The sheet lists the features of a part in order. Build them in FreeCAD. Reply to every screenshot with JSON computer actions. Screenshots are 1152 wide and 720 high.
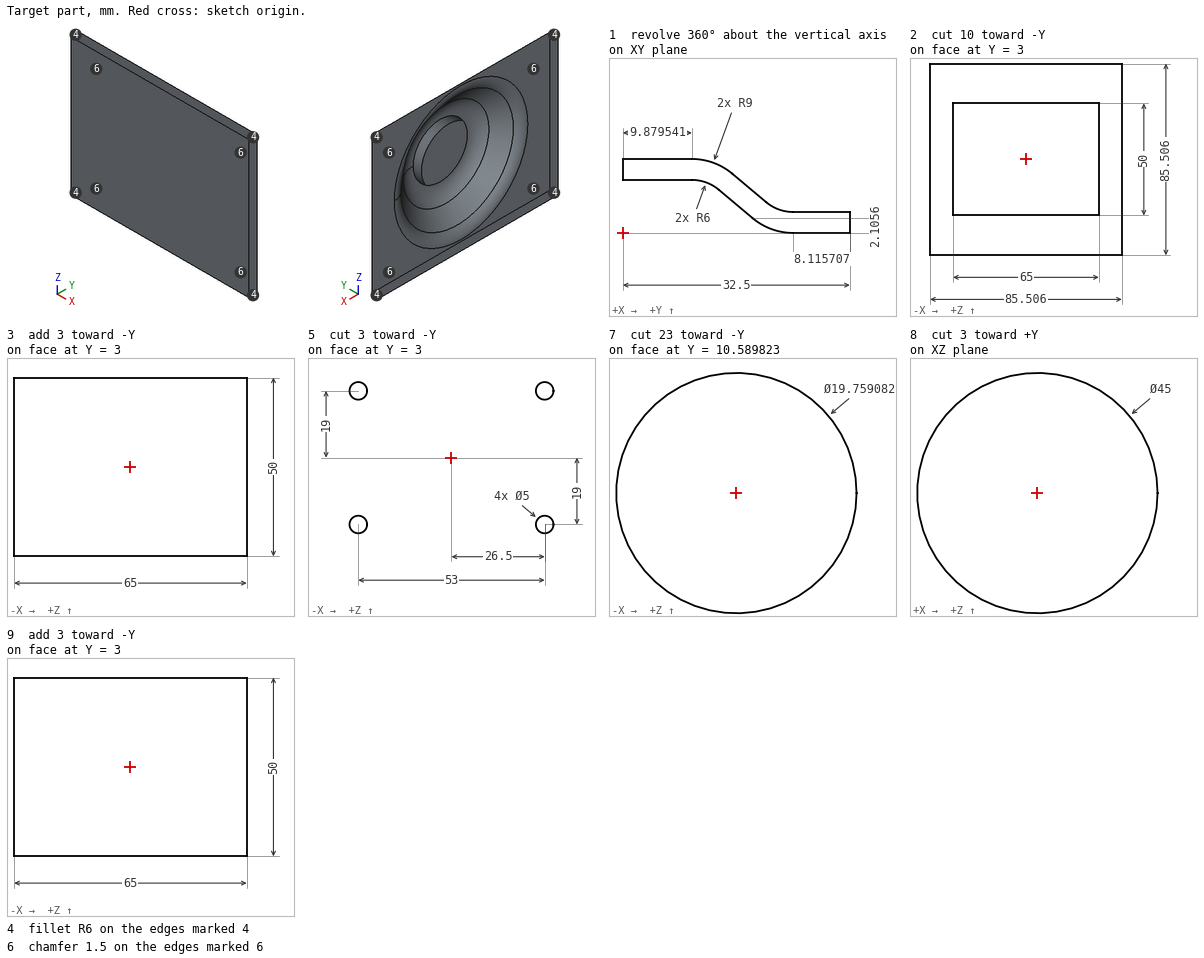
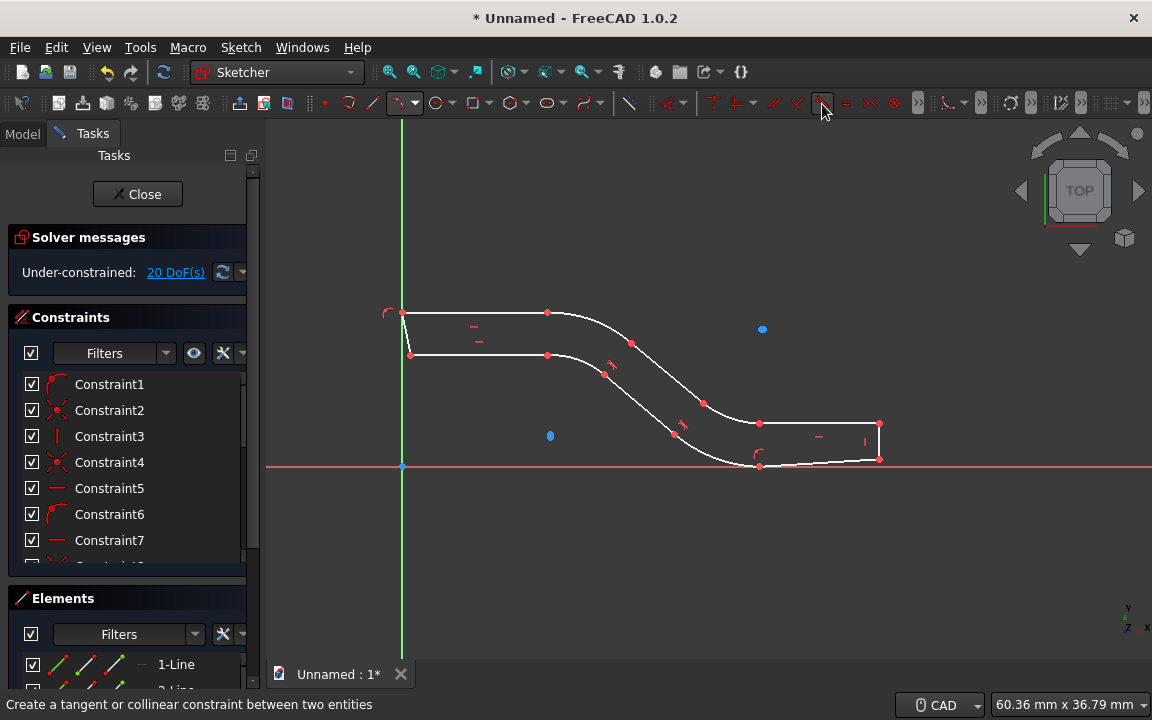
{"action": "left_click", "coordinate": [795, 465]}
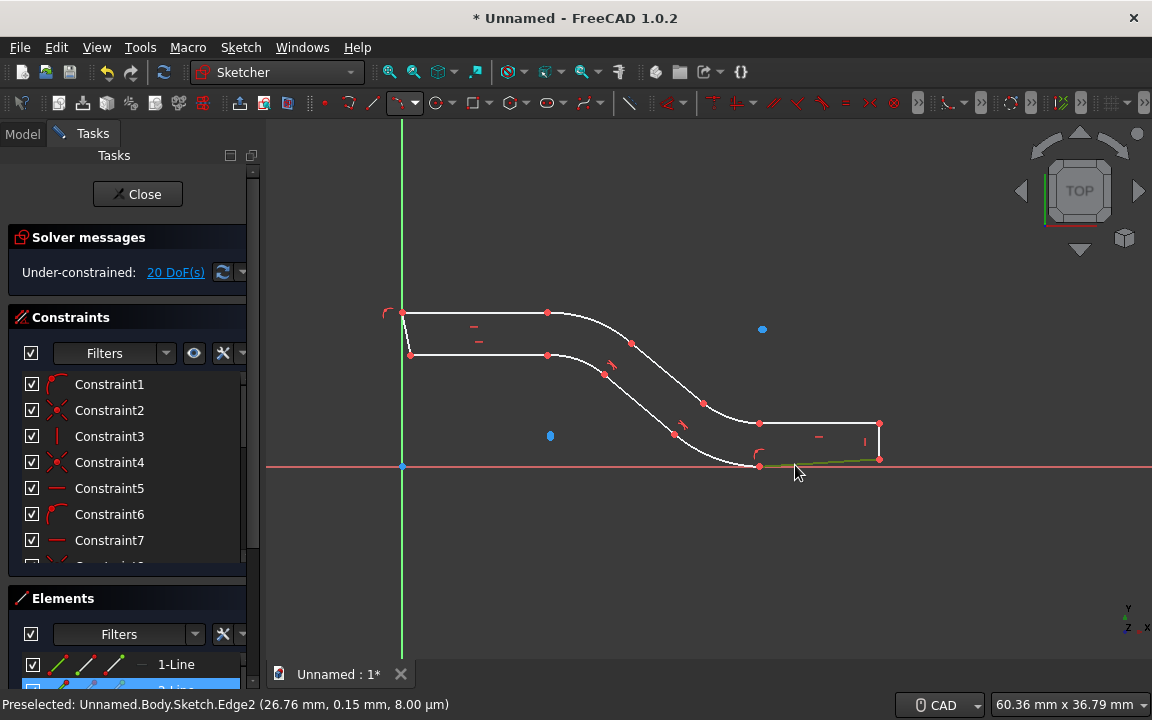
{"action": "left_click", "coordinate": [698, 450]}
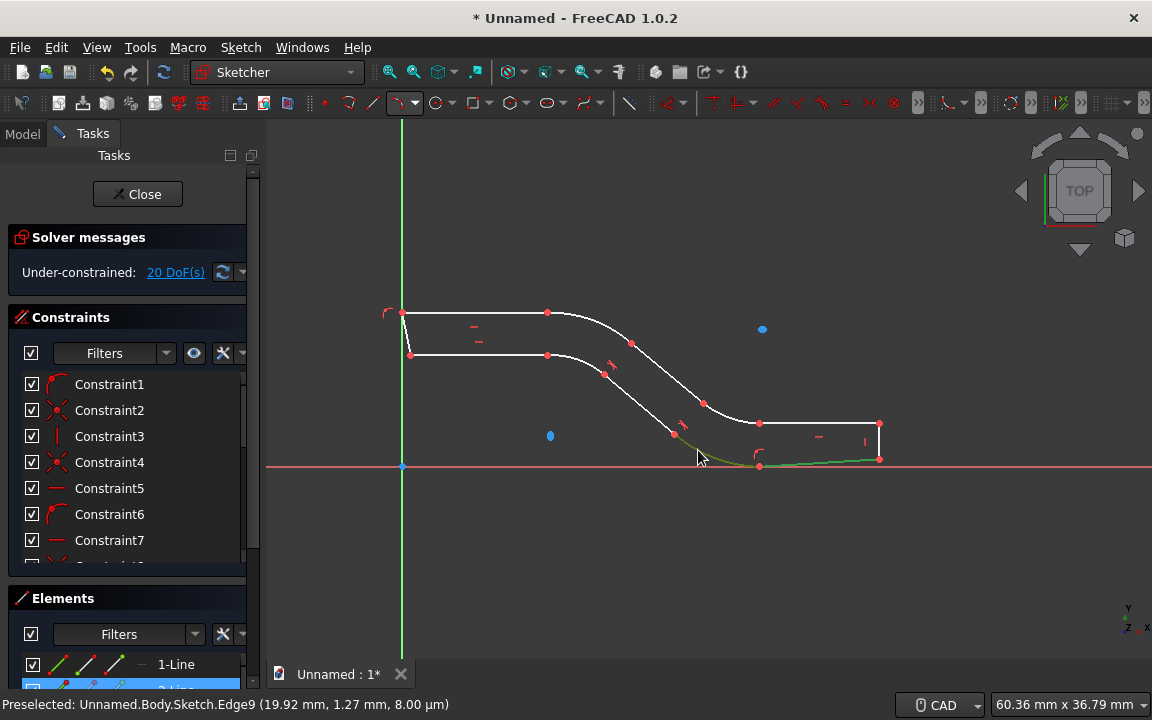
{"action": "left_click", "coordinate": [822, 104]}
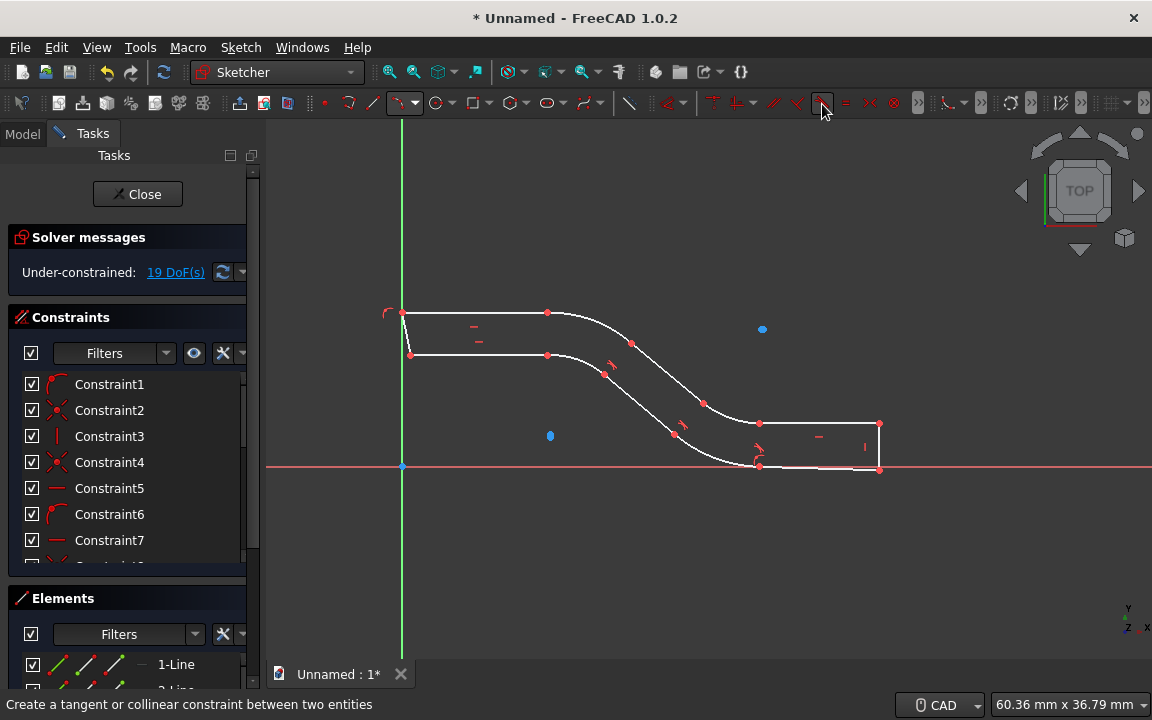
{"action": "left_click", "coordinate": [843, 423]}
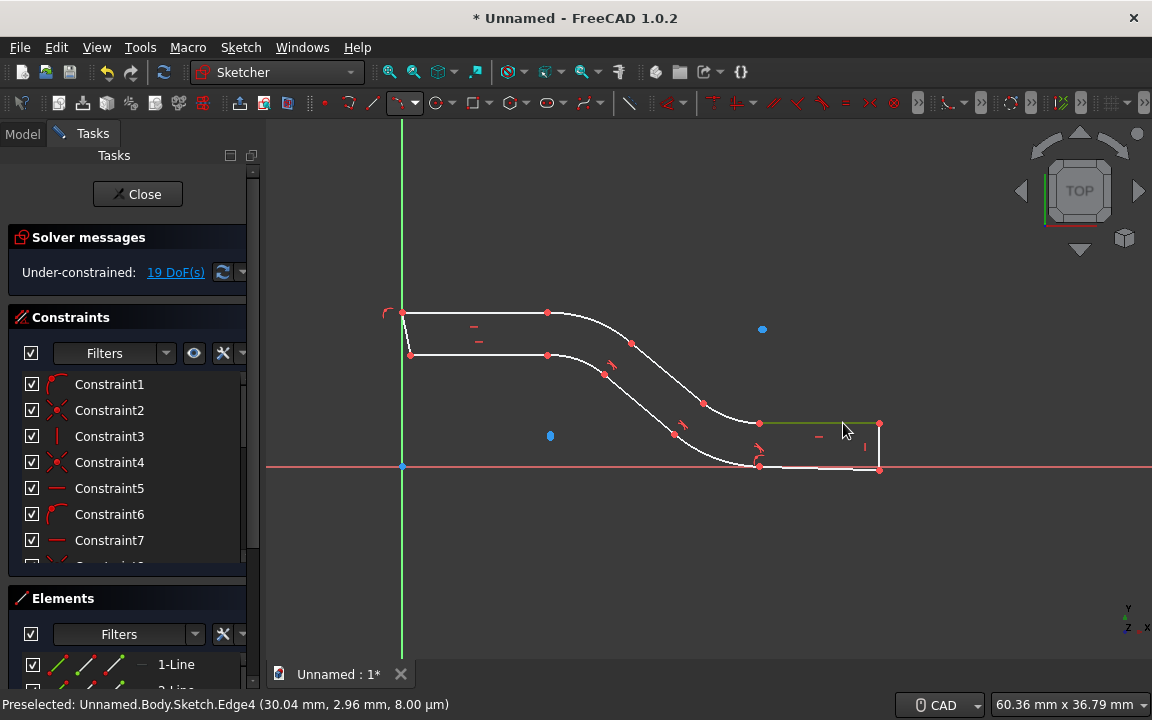
{"action": "left_click", "coordinate": [719, 413]}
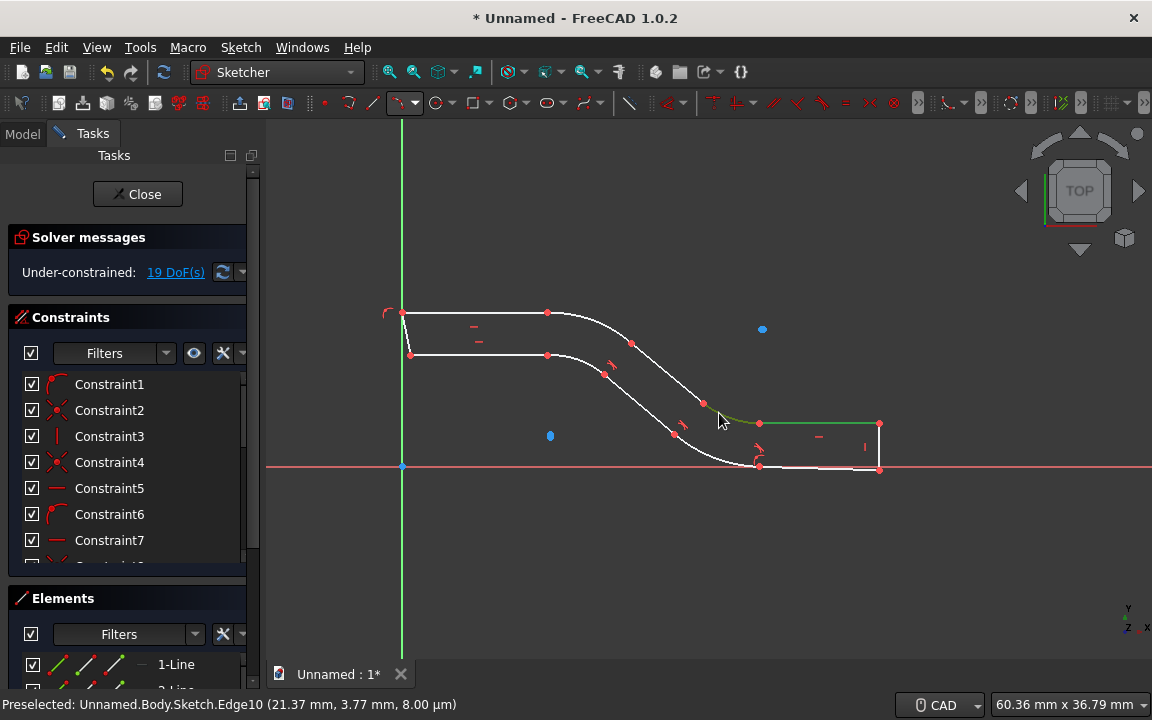
{"action": "left_click", "coordinate": [822, 104]}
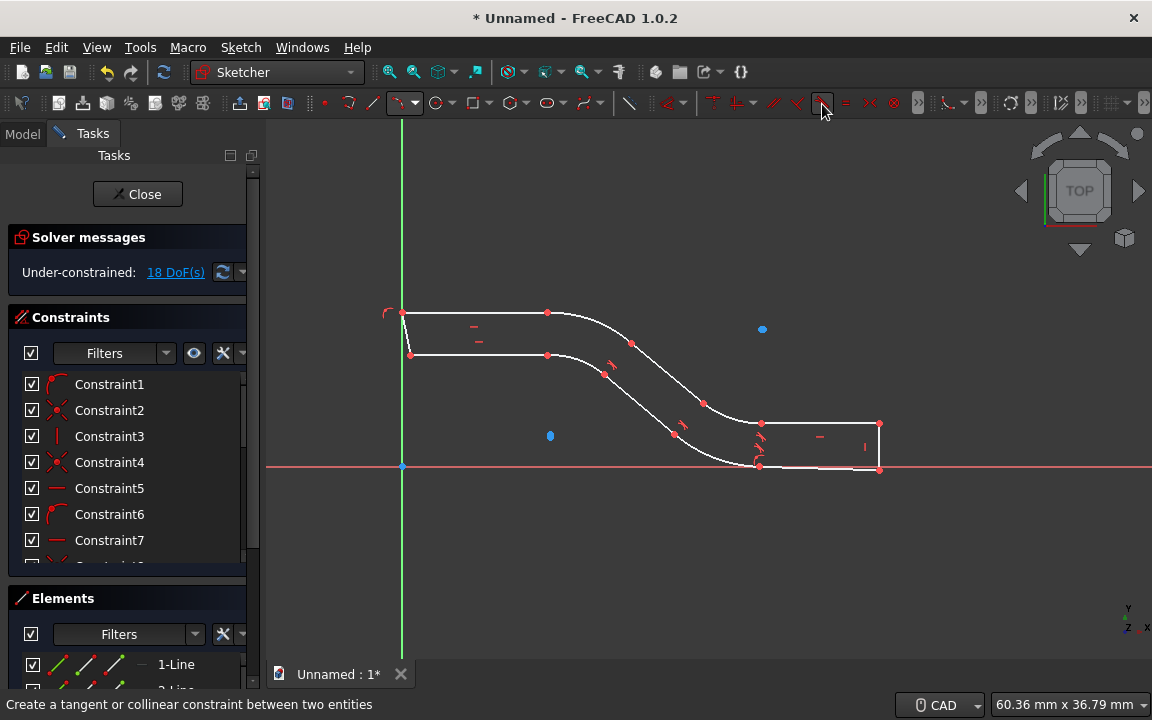
{"action": "left_click", "coordinate": [682, 386]}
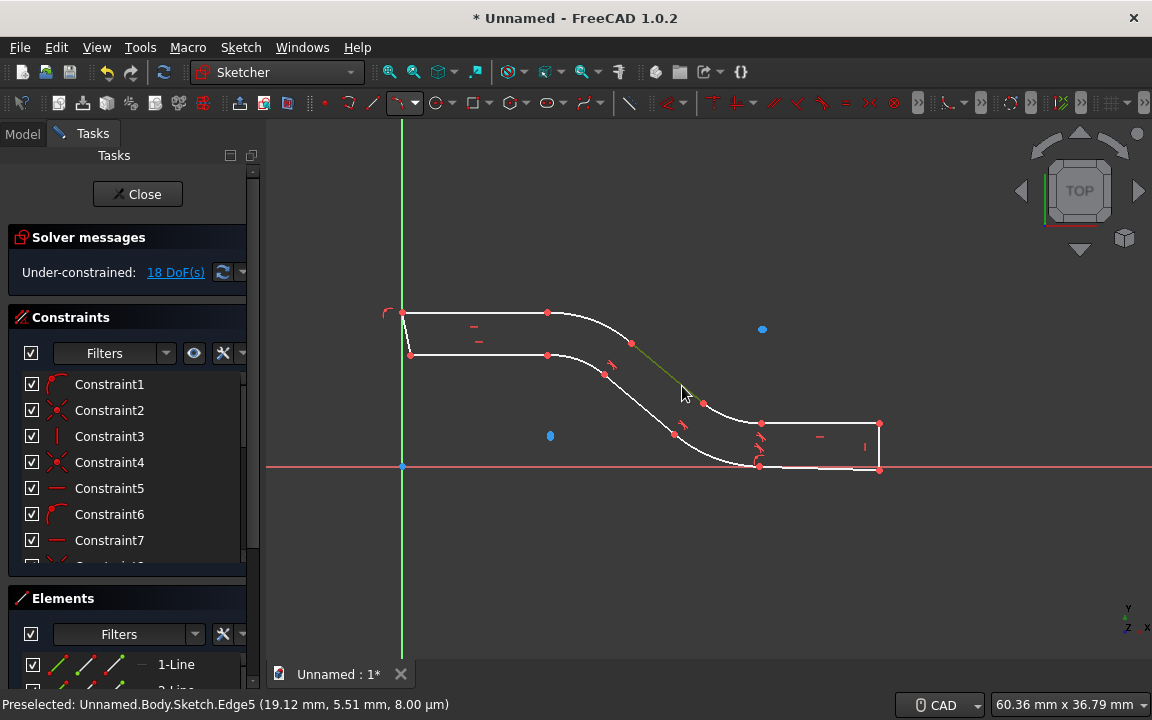
{"action": "left_click", "coordinate": [720, 413]}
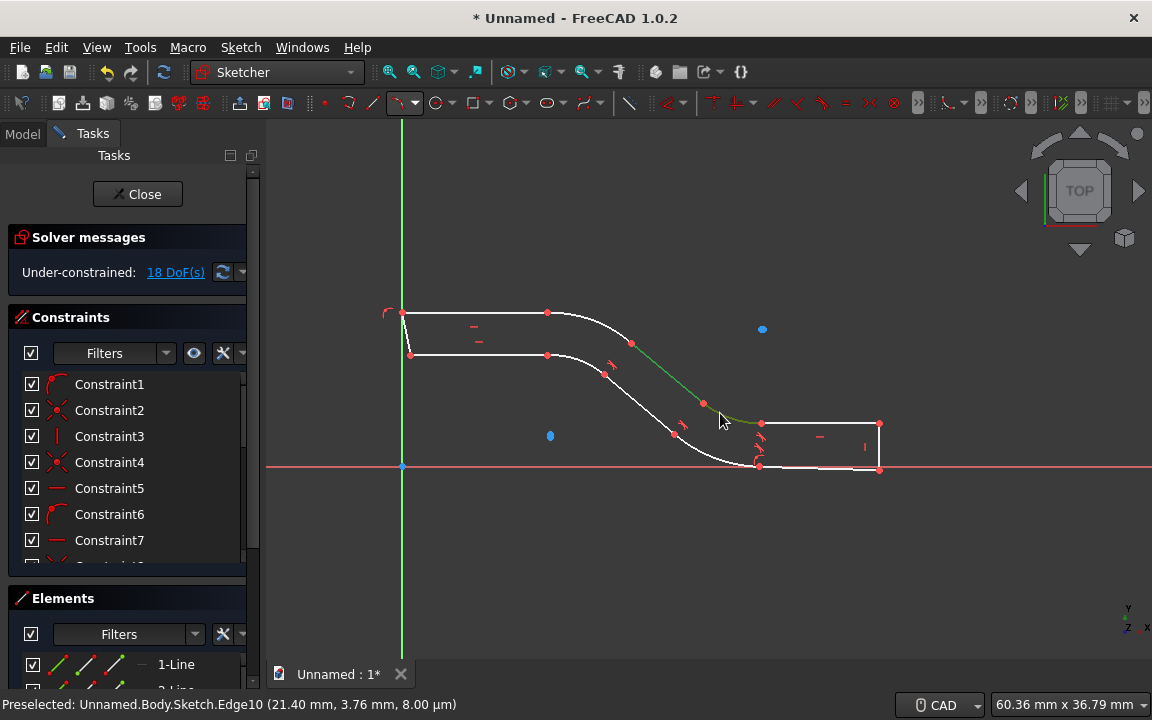
{"action": "left_click", "coordinate": [822, 104]}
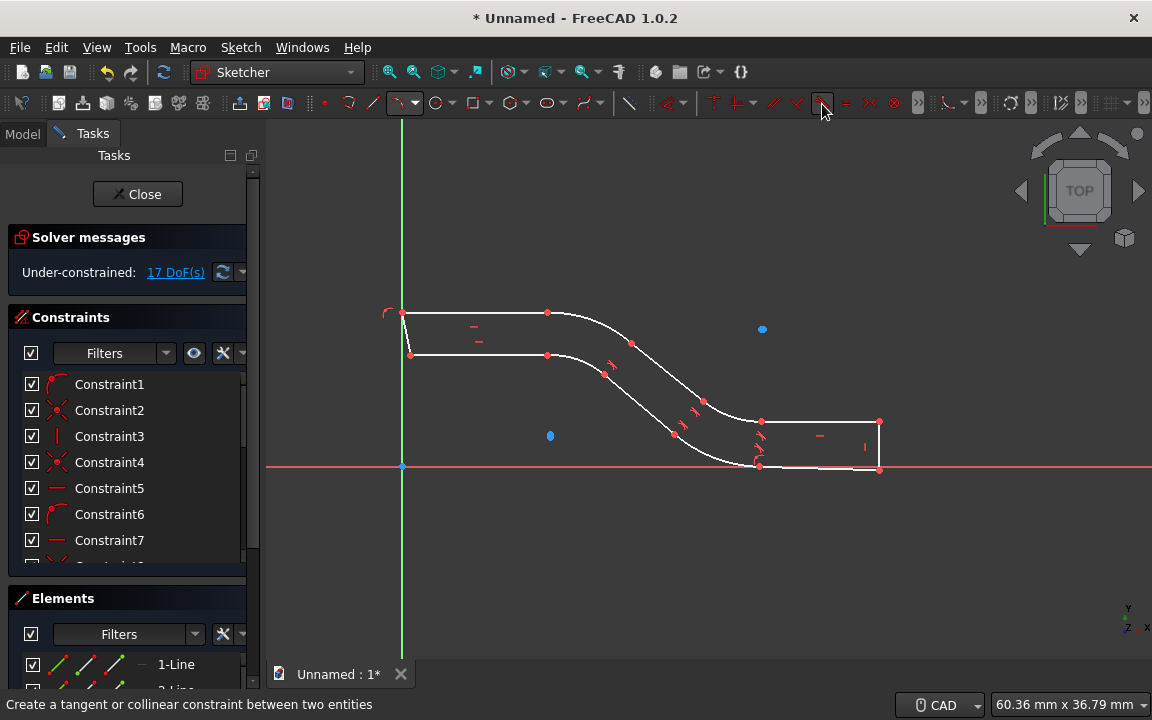
{"action": "left_click", "coordinate": [682, 384]}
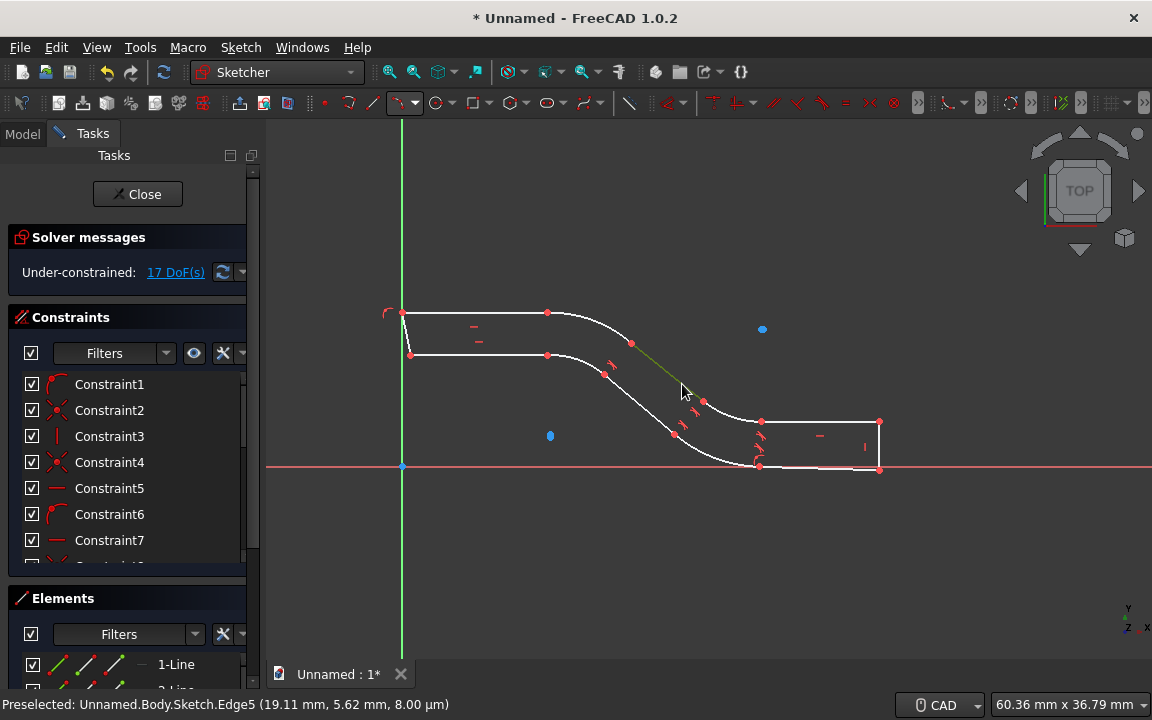
{"action": "left_click", "coordinate": [609, 328]}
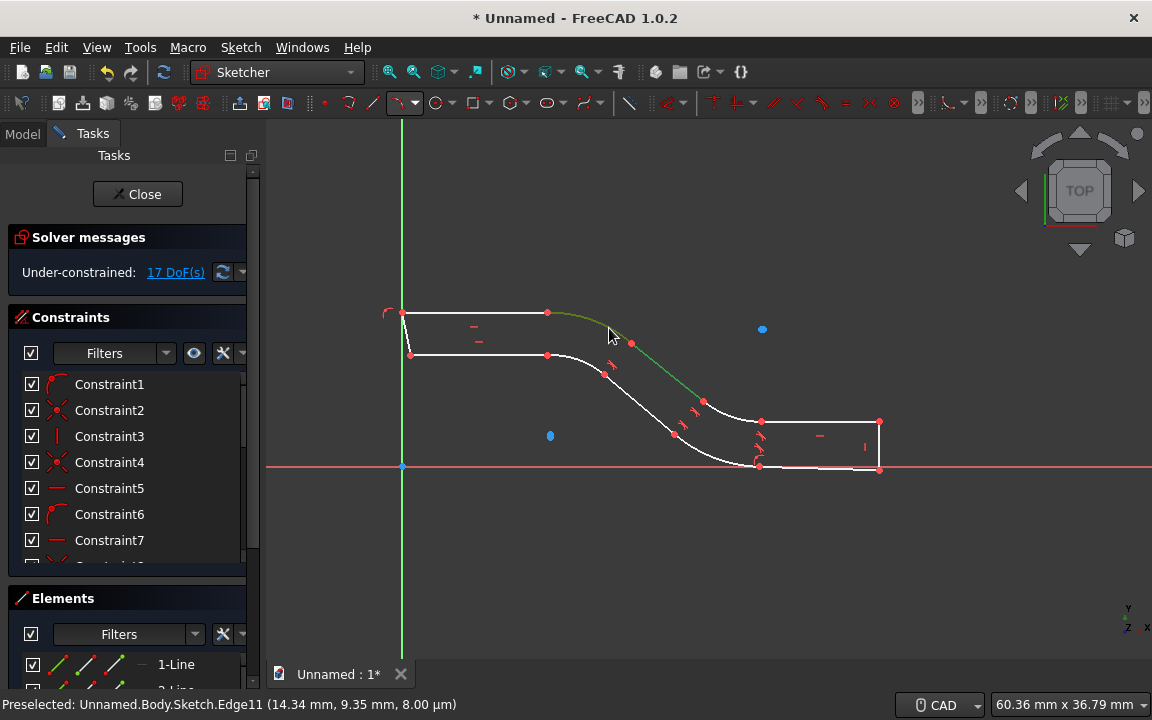
{"action": "left_click", "coordinate": [822, 104]}